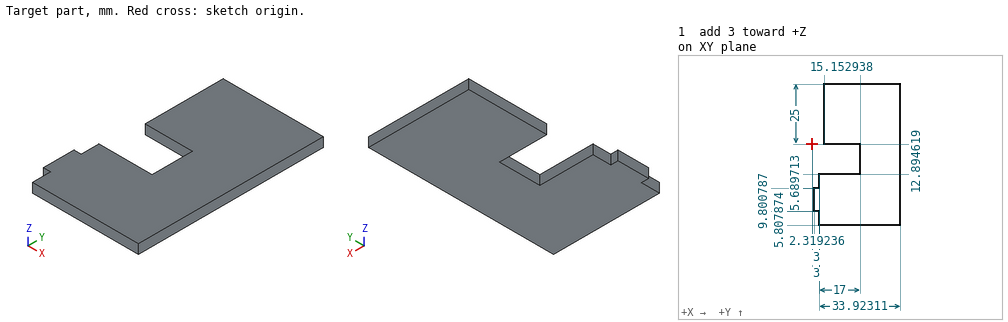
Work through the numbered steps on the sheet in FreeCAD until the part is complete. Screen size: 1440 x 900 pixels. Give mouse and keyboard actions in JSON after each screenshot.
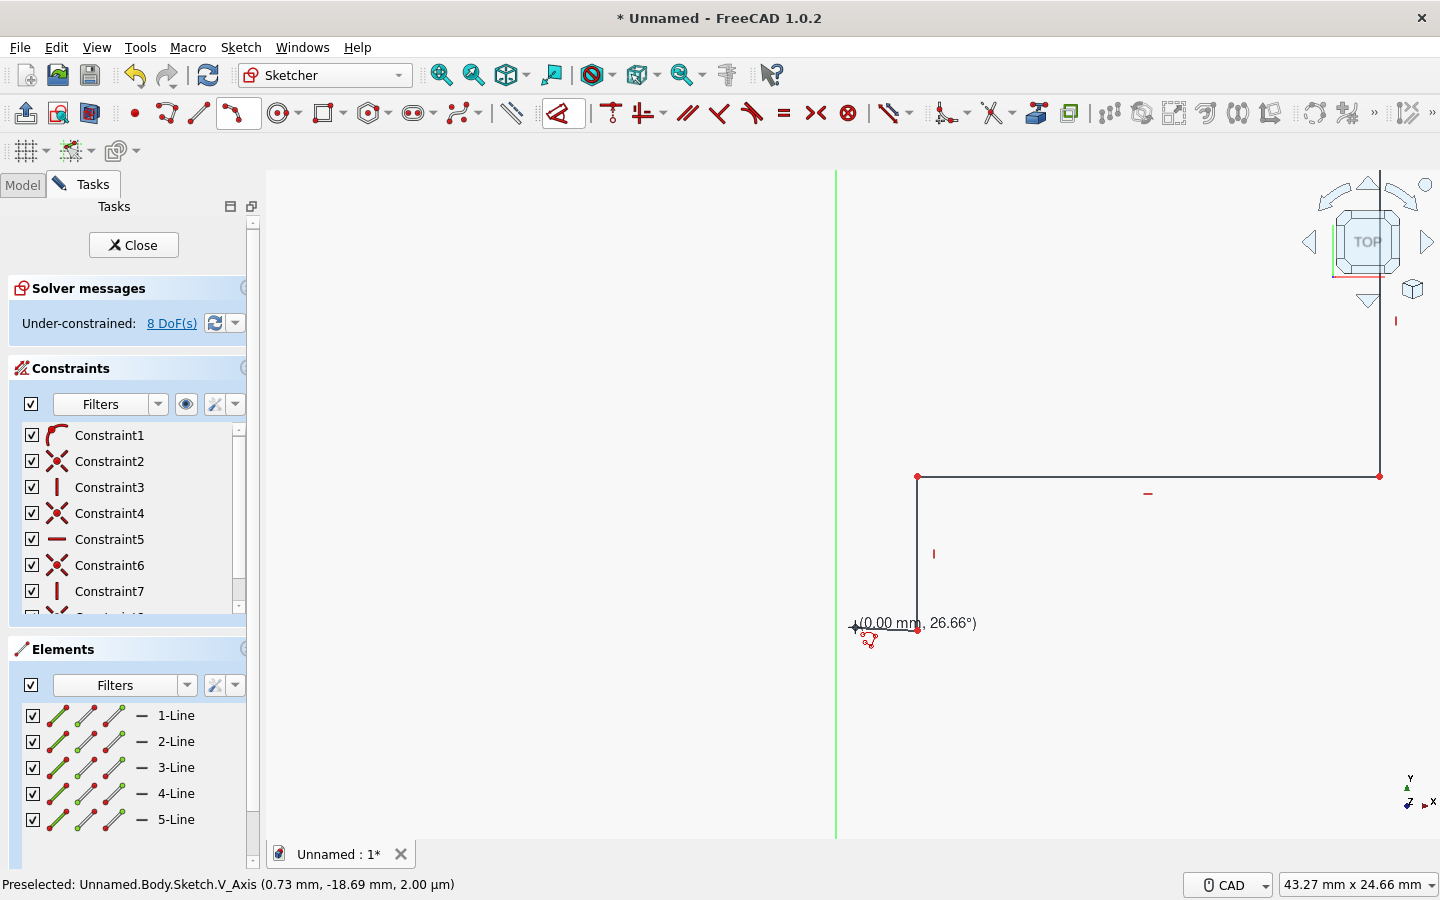
{"action": "scroll", "coordinate": [604, 589], "scroll_direction": "down", "scroll_amount": 7}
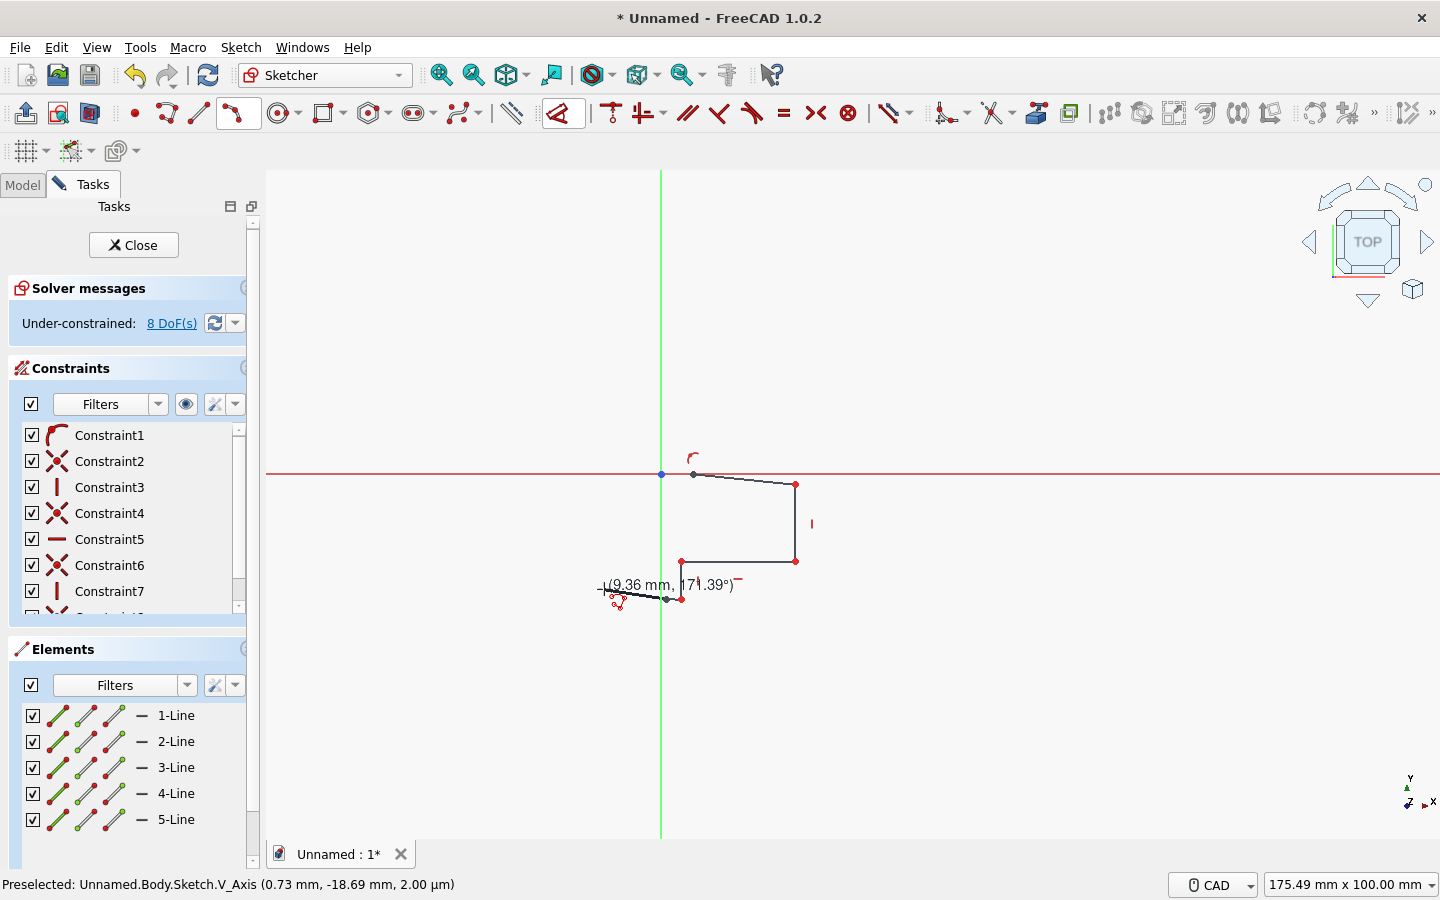
{"action": "scroll", "coordinate": [666, 664], "scroll_direction": "up", "scroll_amount": 7}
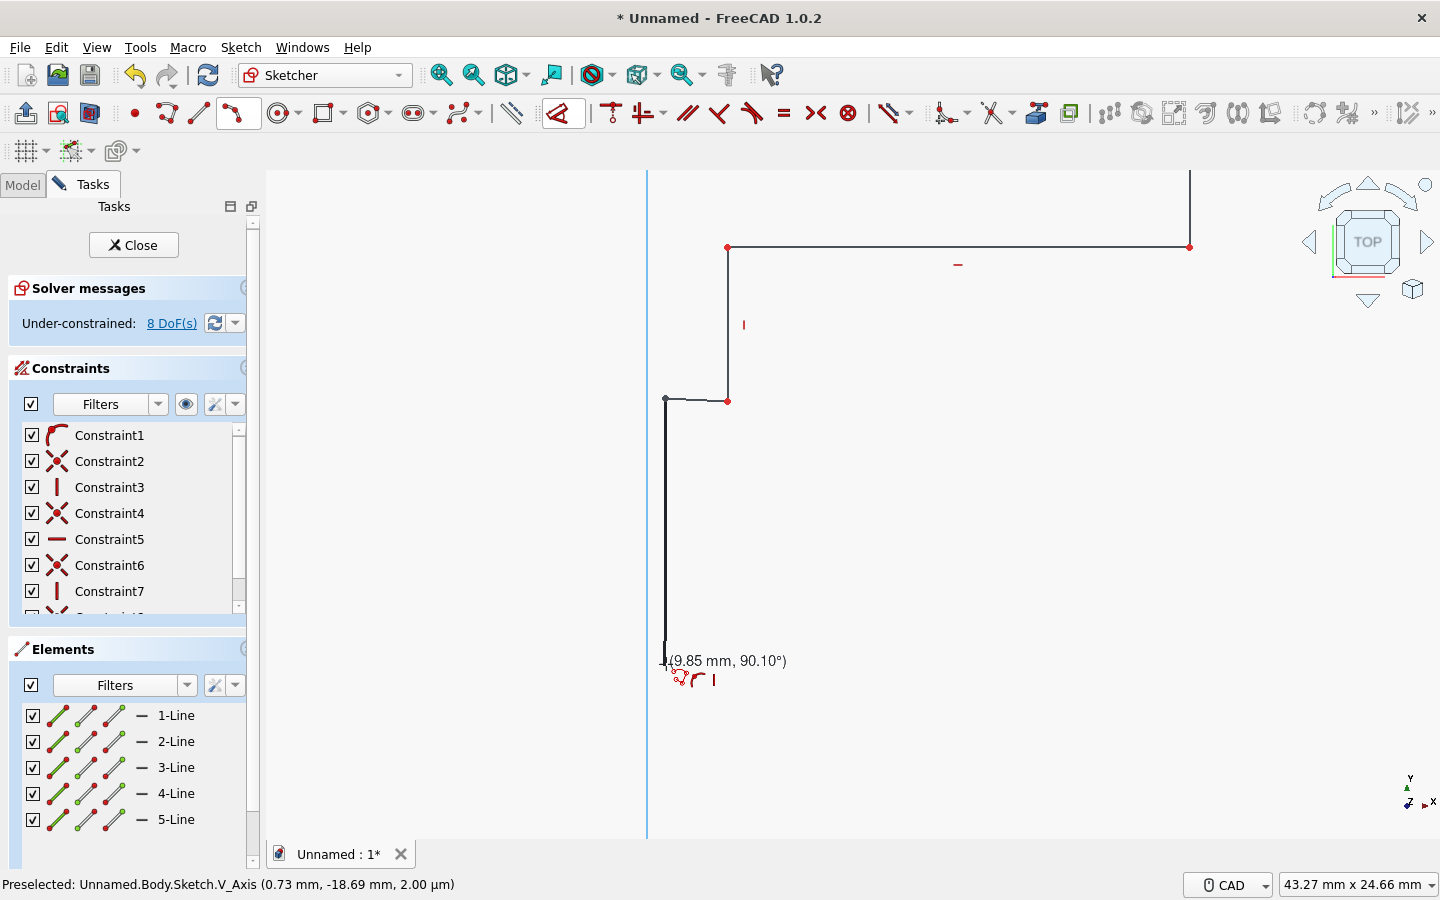
{"action": "left_click", "coordinate": [665, 663]}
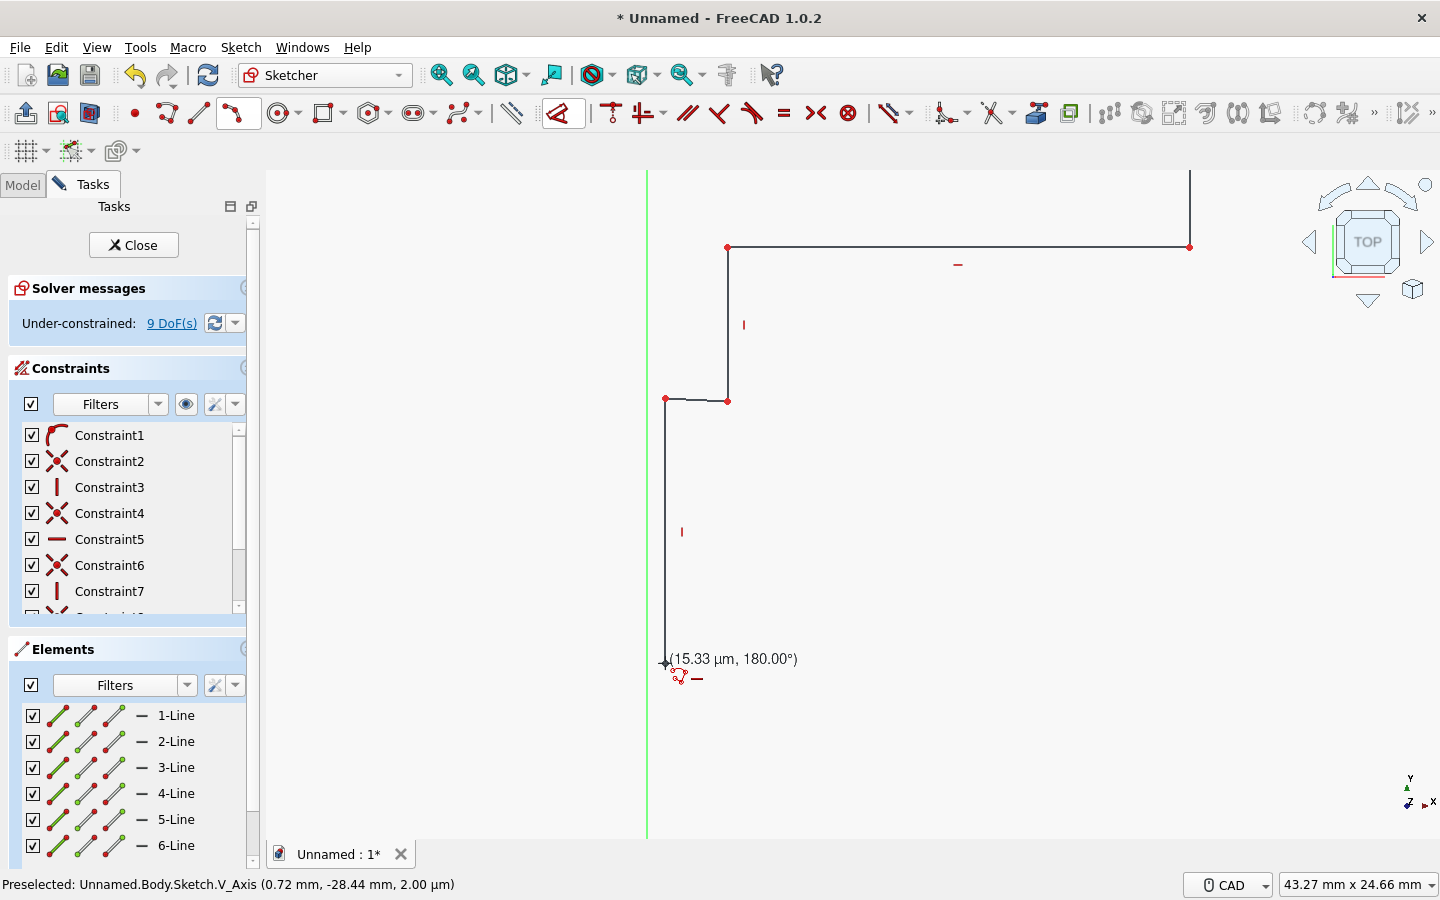
{"action": "scroll", "coordinate": [666, 664], "scroll_direction": "down", "scroll_amount": 7}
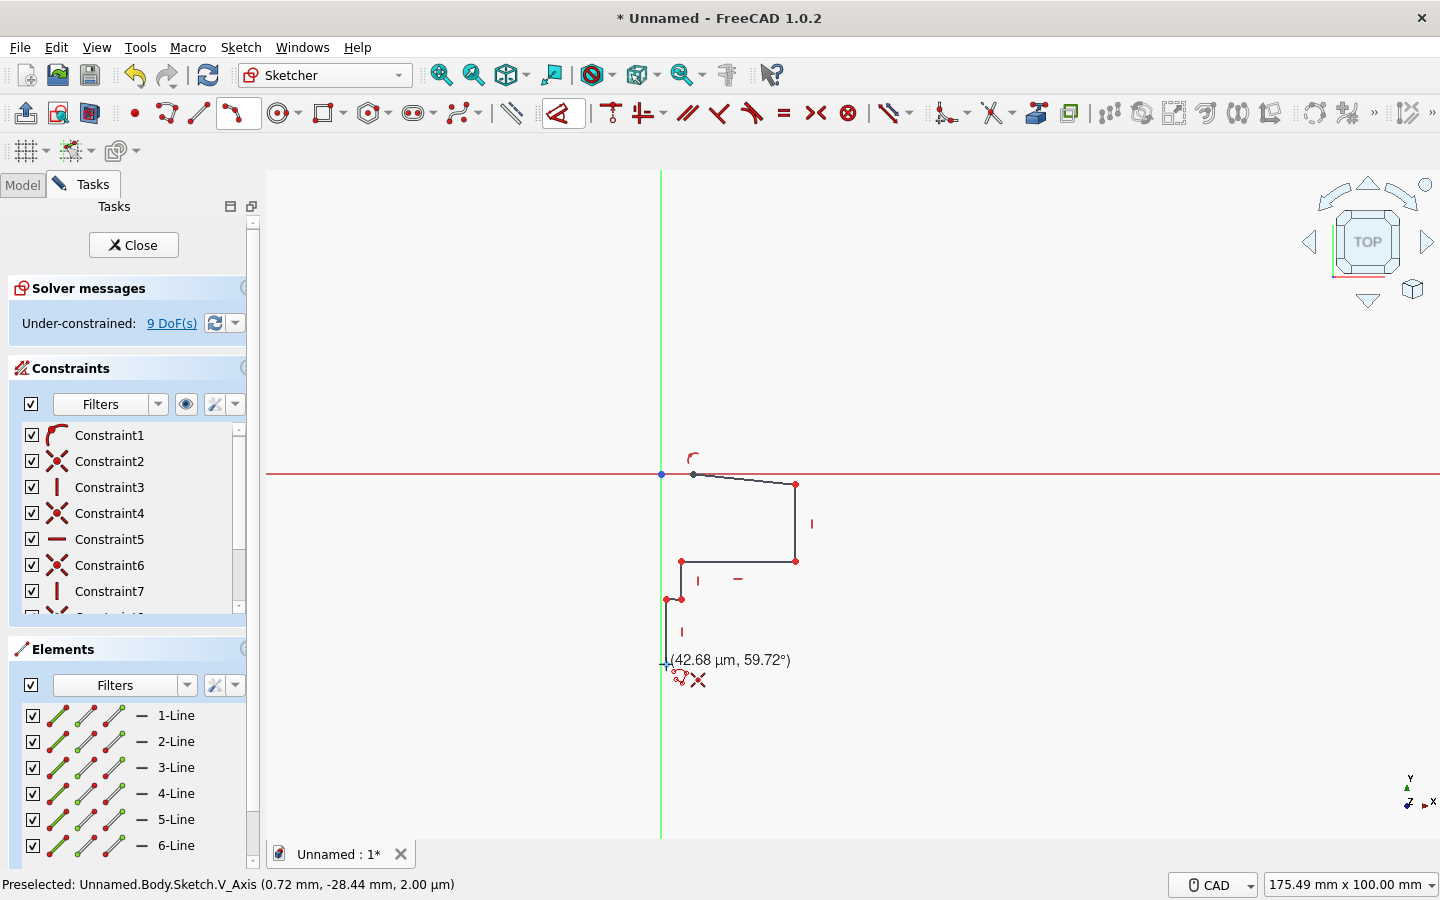
{"action": "left_click", "coordinate": [682, 664]}
{"action": "left_click", "coordinate": [682, 703]}
{"action": "left_click", "coordinate": [908, 703]}
{"action": "left_click", "coordinate": [908, 307]}
{"action": "left_click", "coordinate": [694, 307]}
{"action": "left_click", "coordinate": [693, 474]}
{"action": "key", "text": "Escape"}
{"action": "key", "text": "Escape"}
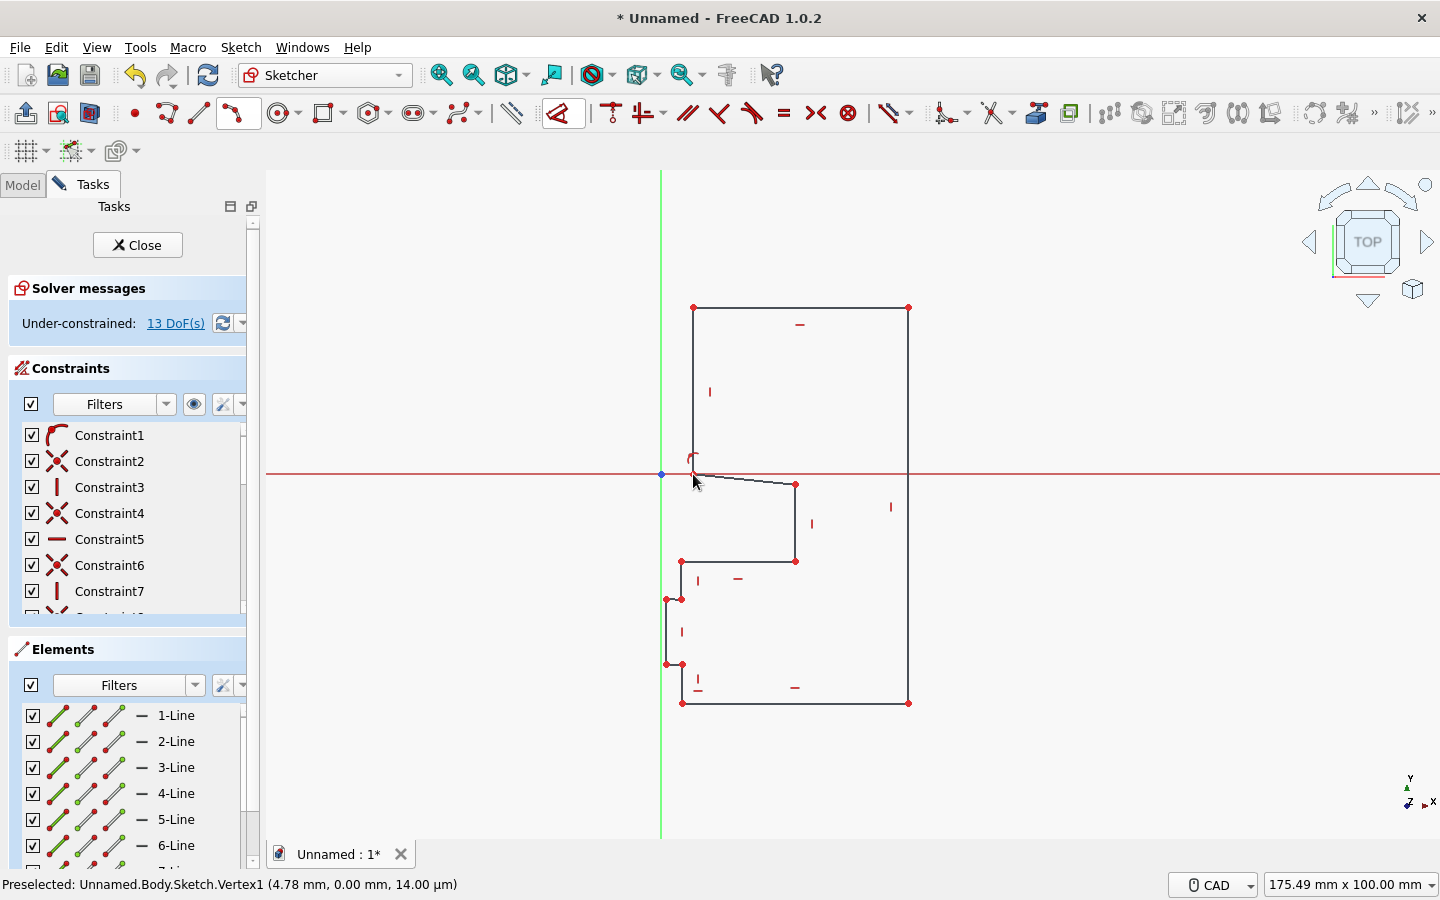
{"action": "left_click", "coordinate": [724, 477]}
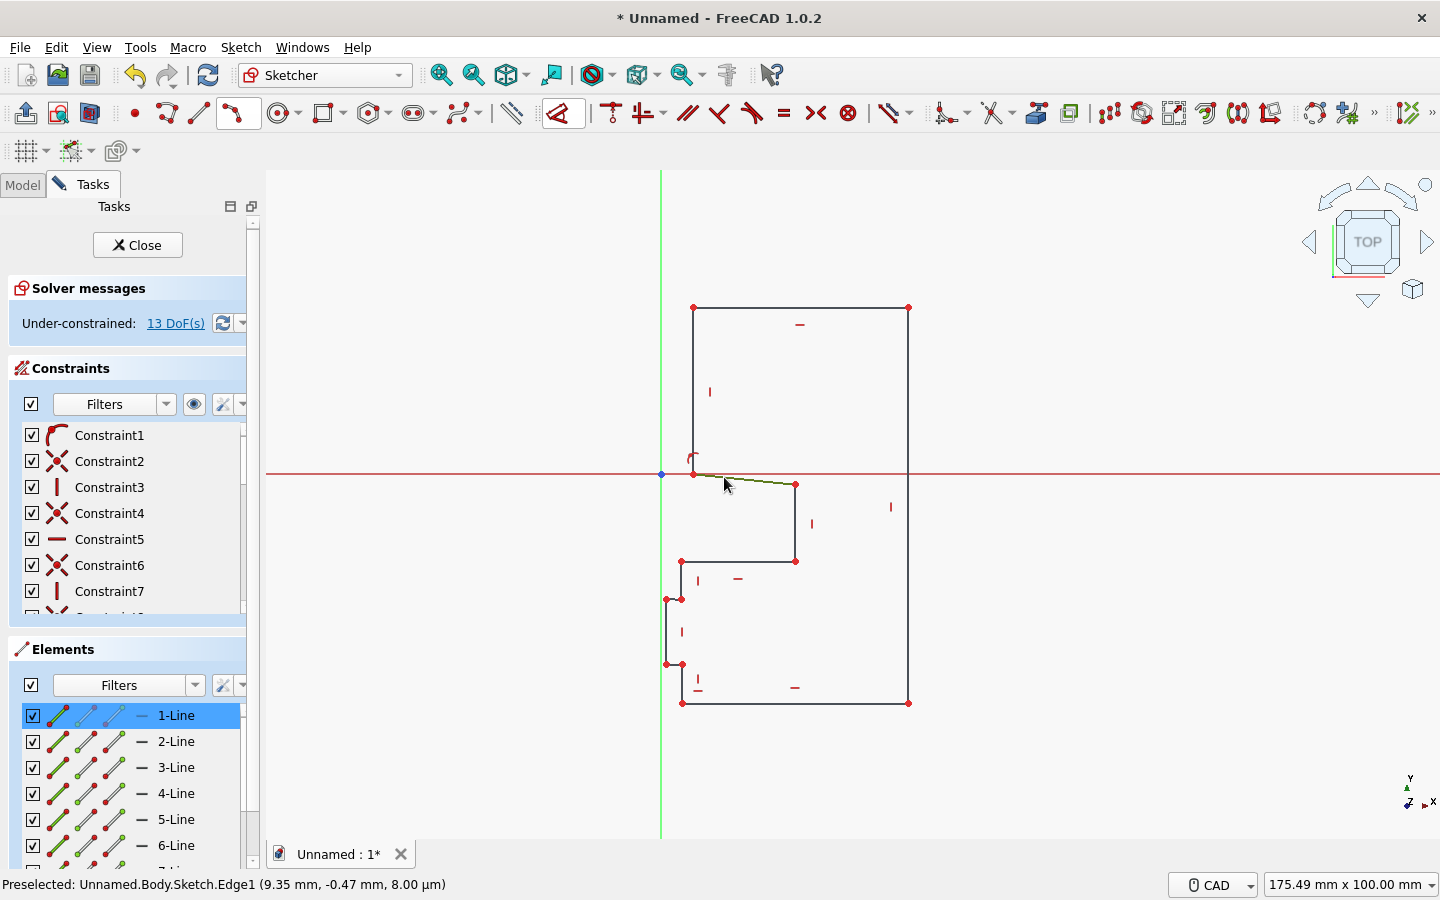
{"action": "key", "text": "h"}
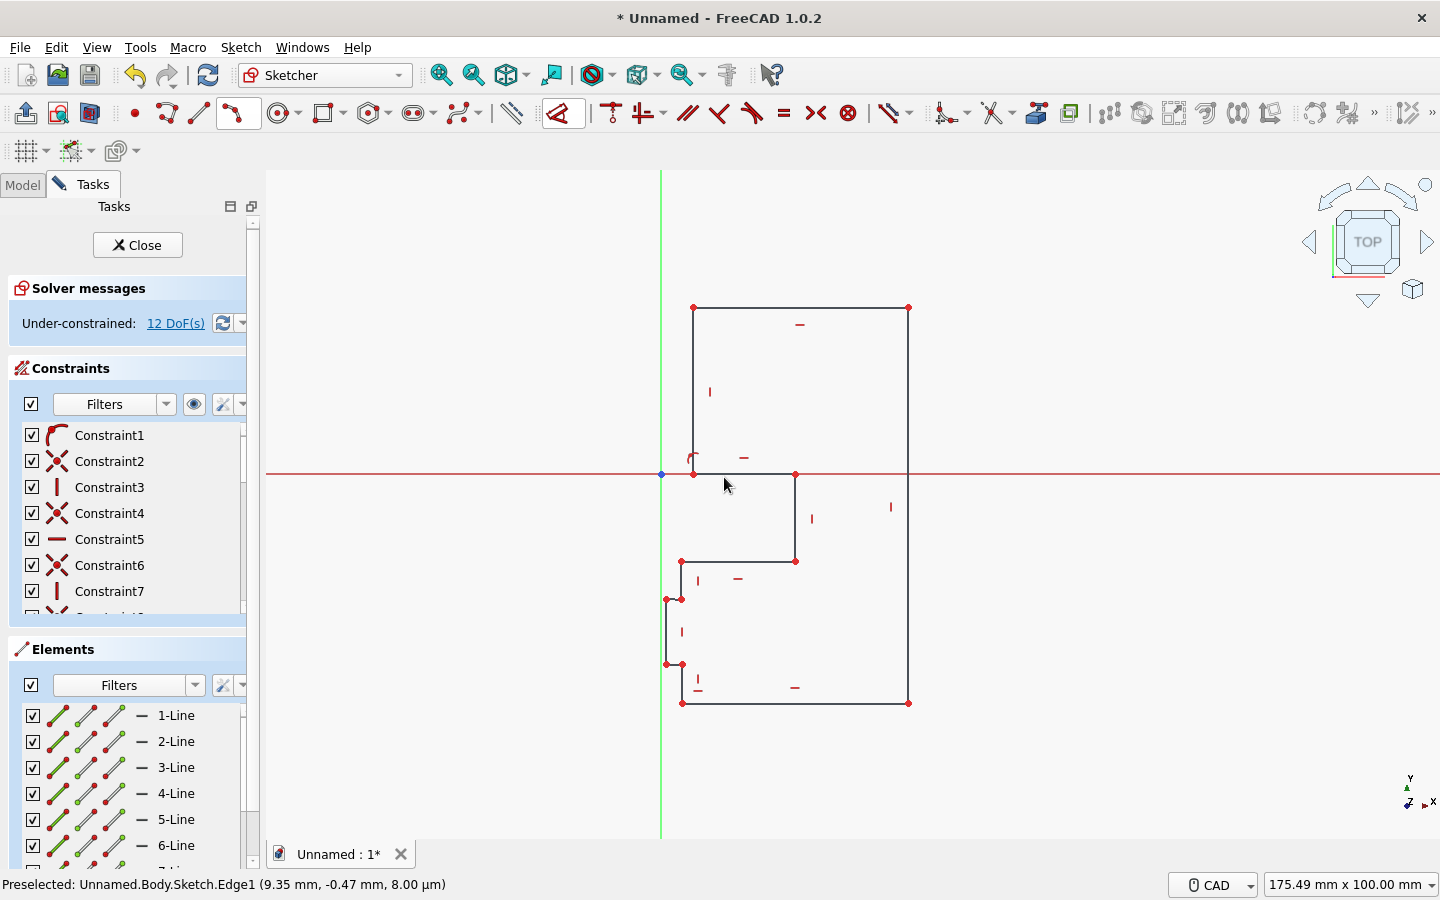
{"action": "scroll", "coordinate": [674, 599], "scroll_direction": "up", "scroll_amount": 3}